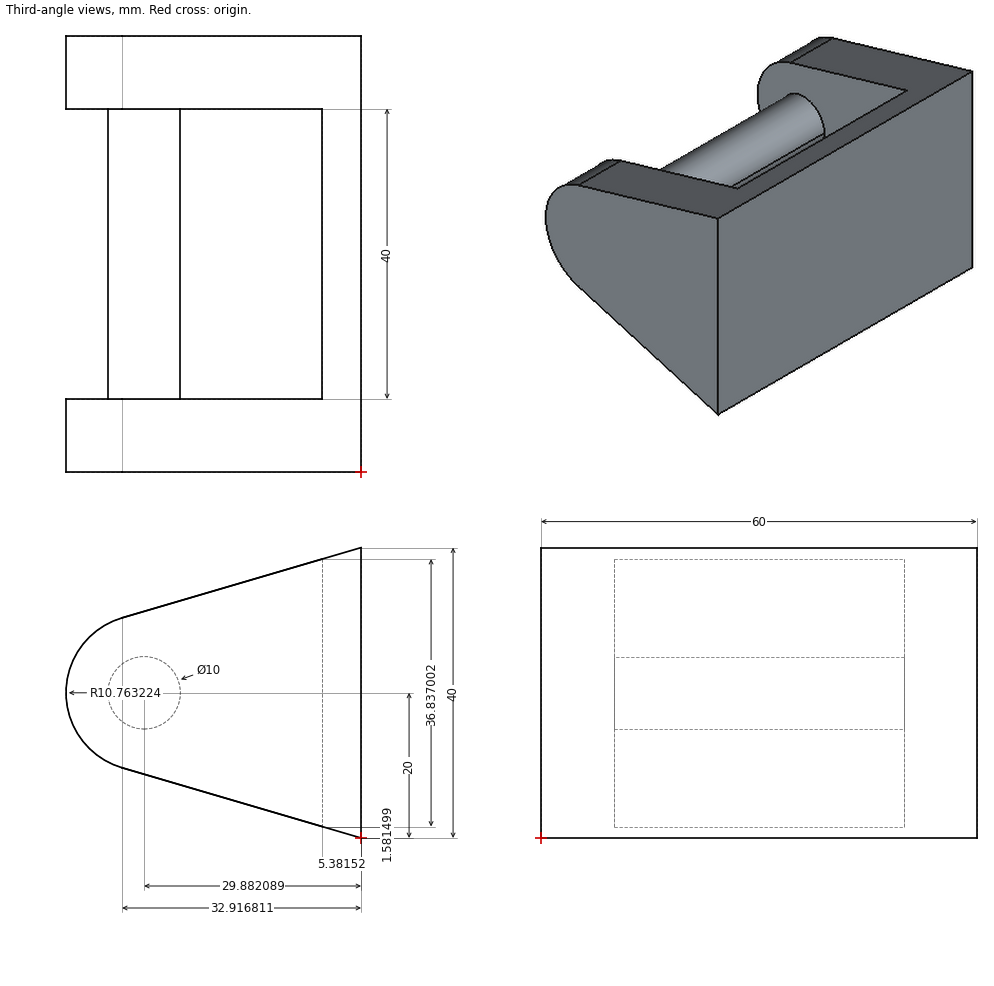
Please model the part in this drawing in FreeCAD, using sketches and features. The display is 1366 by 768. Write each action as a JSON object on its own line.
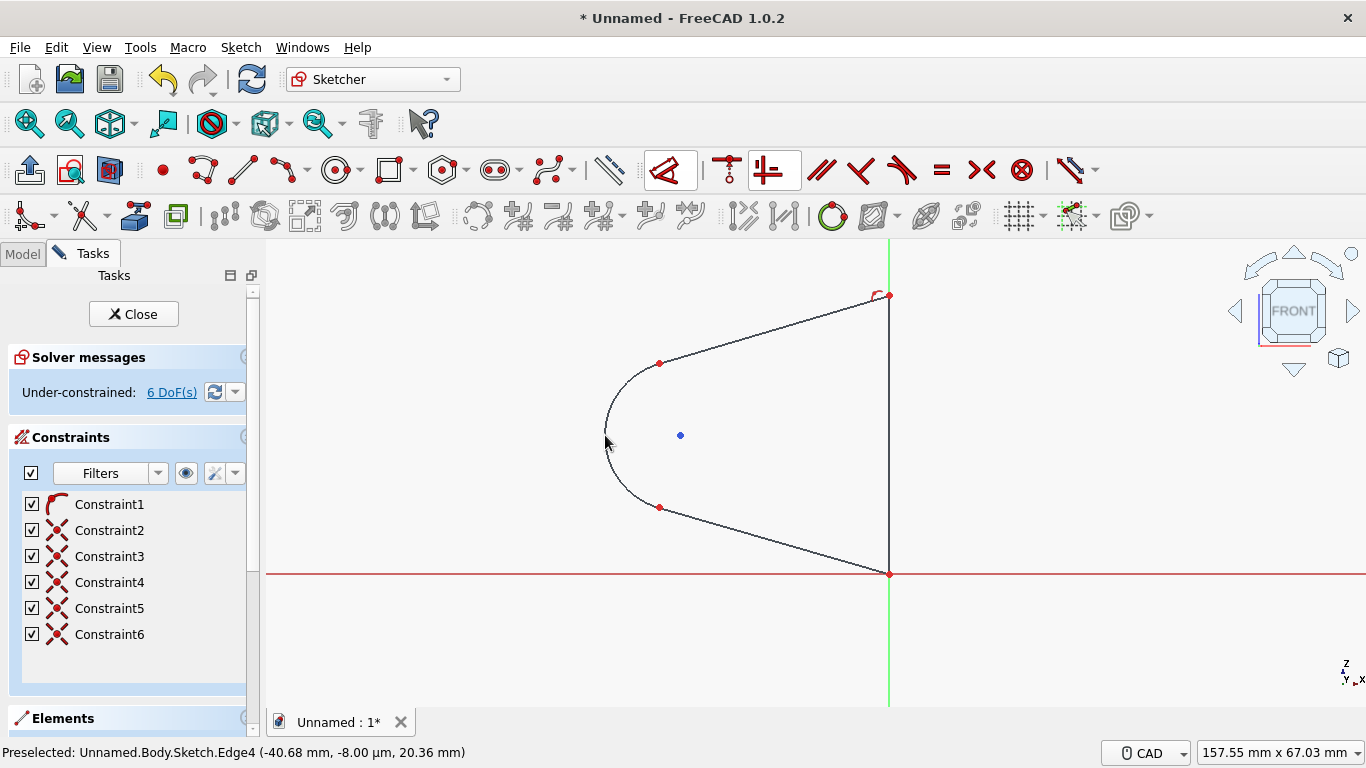
{"action": "left_click", "coordinate": [728, 344]}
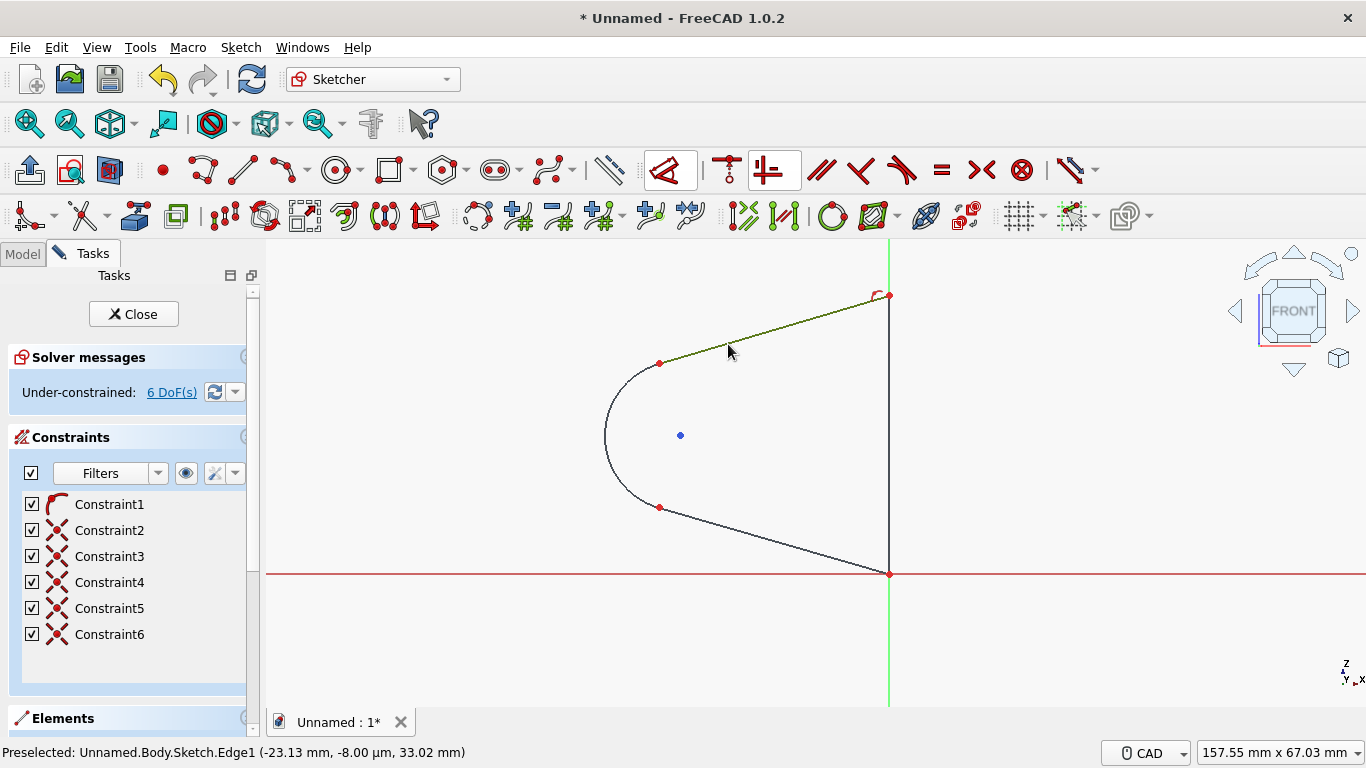
{"action": "left_click", "coordinate": [615, 399]}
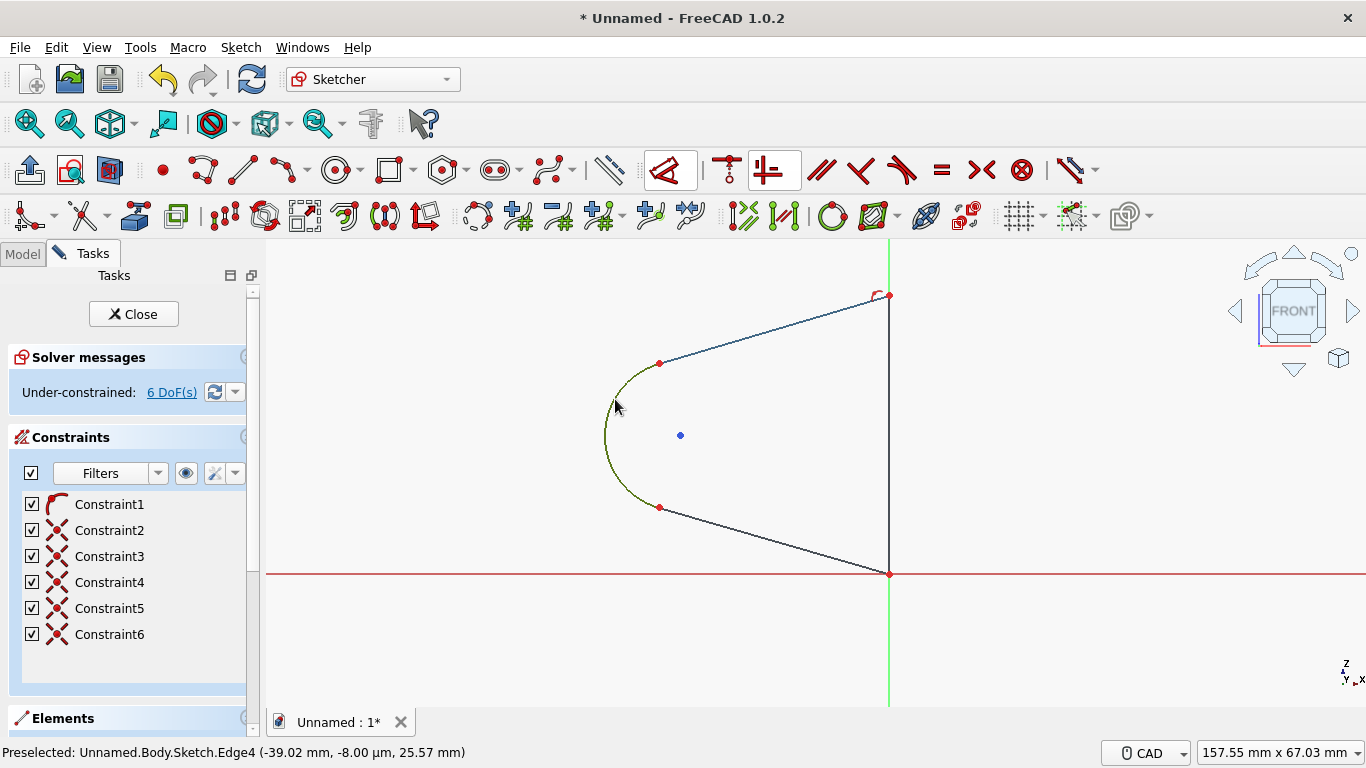
{"action": "left_click", "coordinate": [902, 170]}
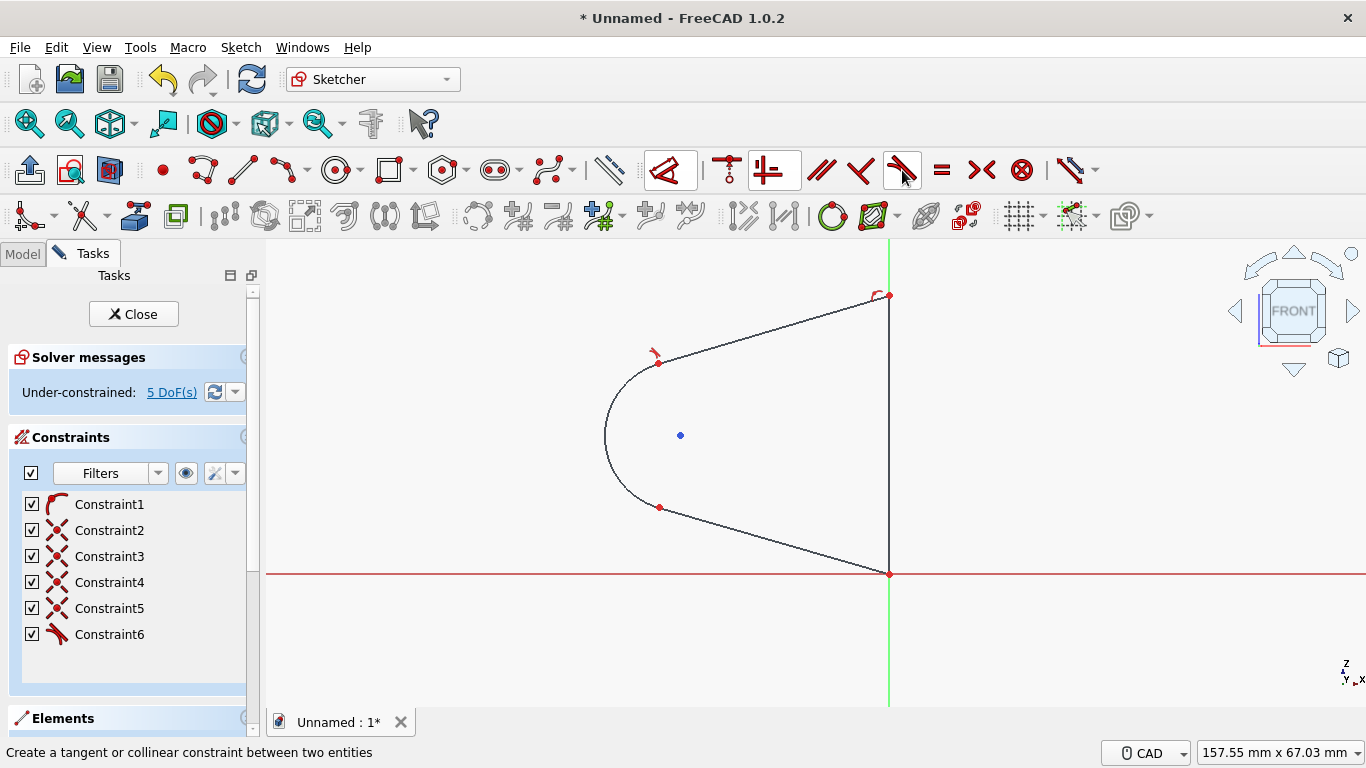
{"action": "left_click", "coordinate": [820, 554]}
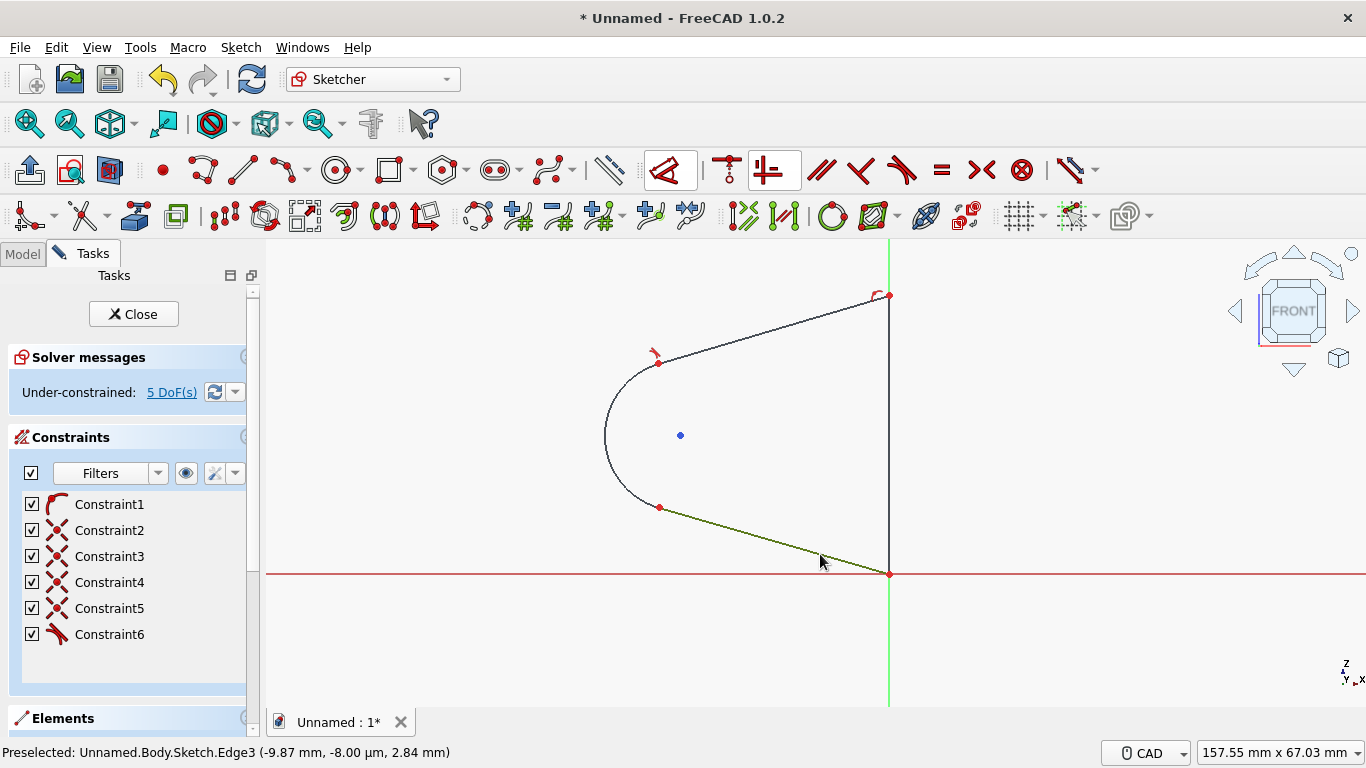
{"action": "left_click", "coordinate": [615, 399]}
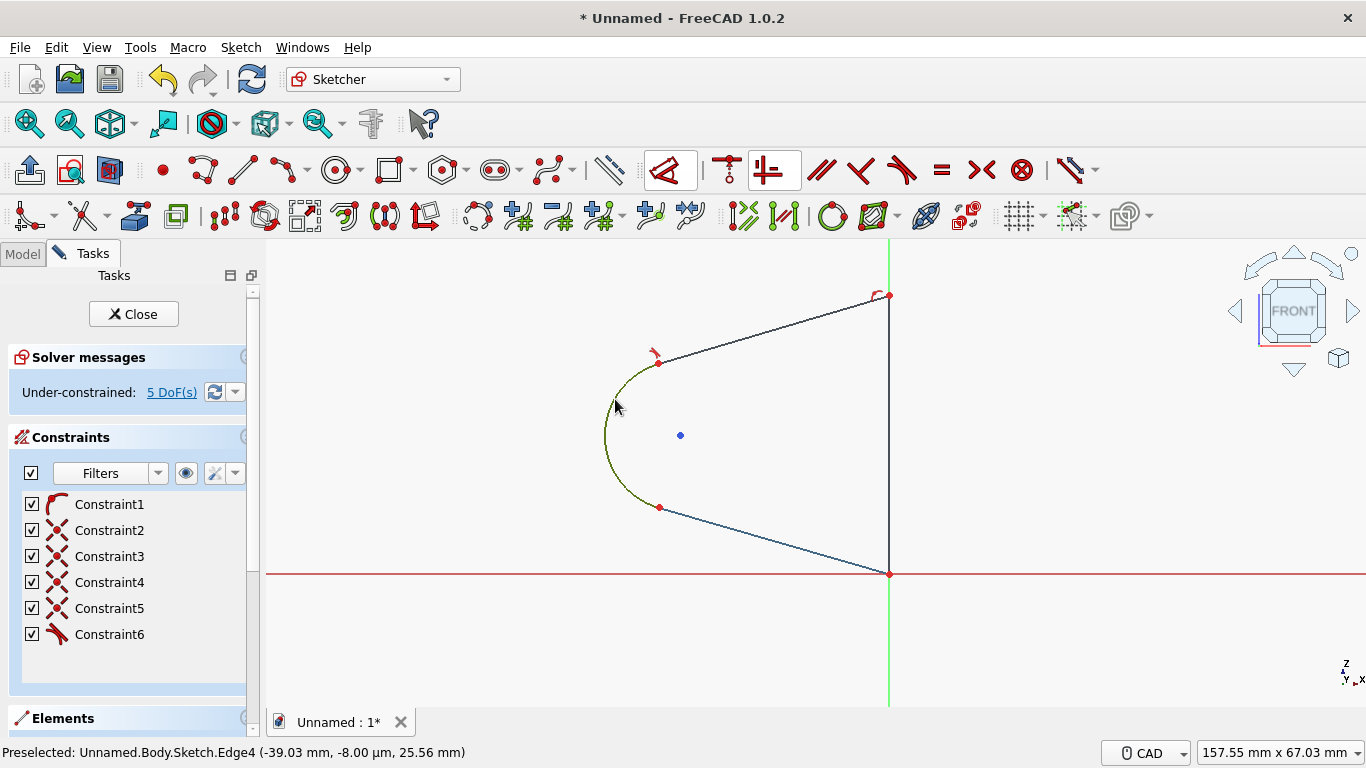
{"action": "left_click", "coordinate": [902, 170]}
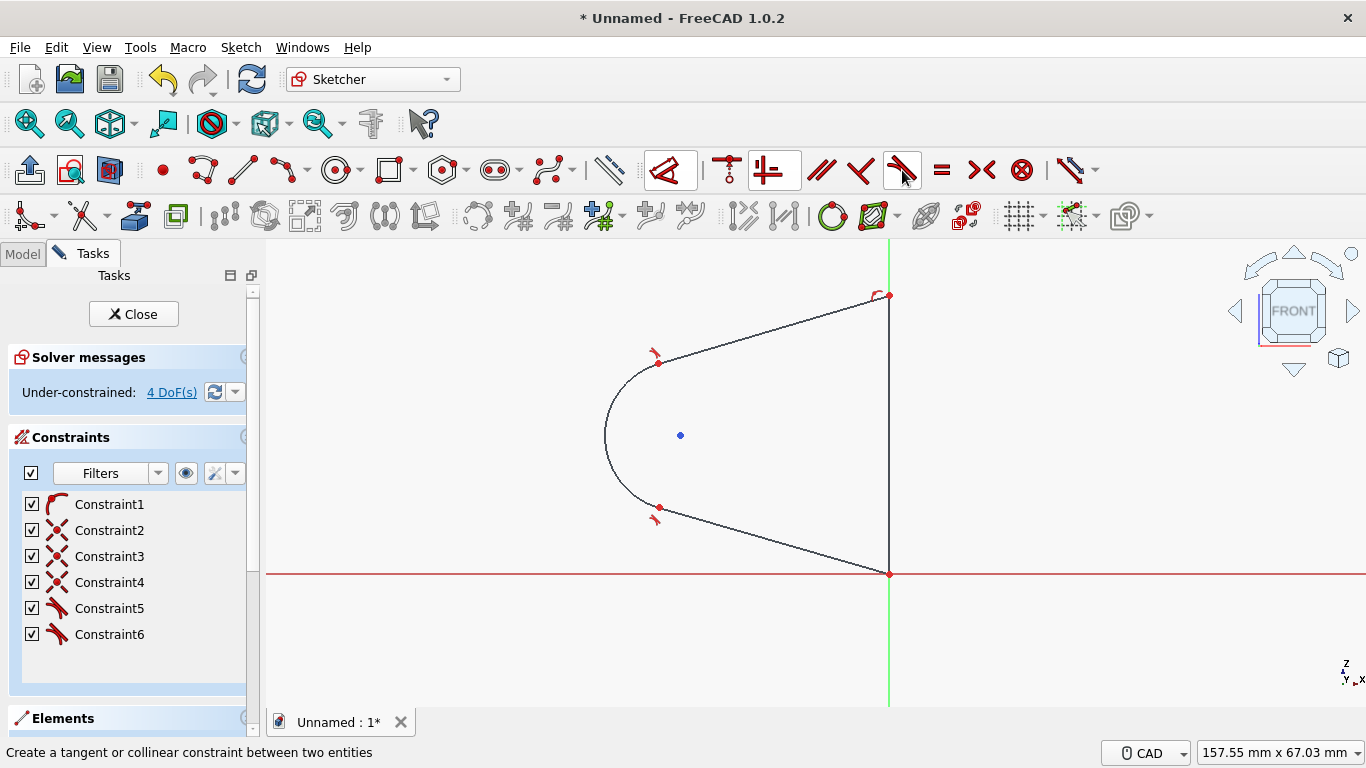
{"action": "left_click", "coordinate": [664, 170]}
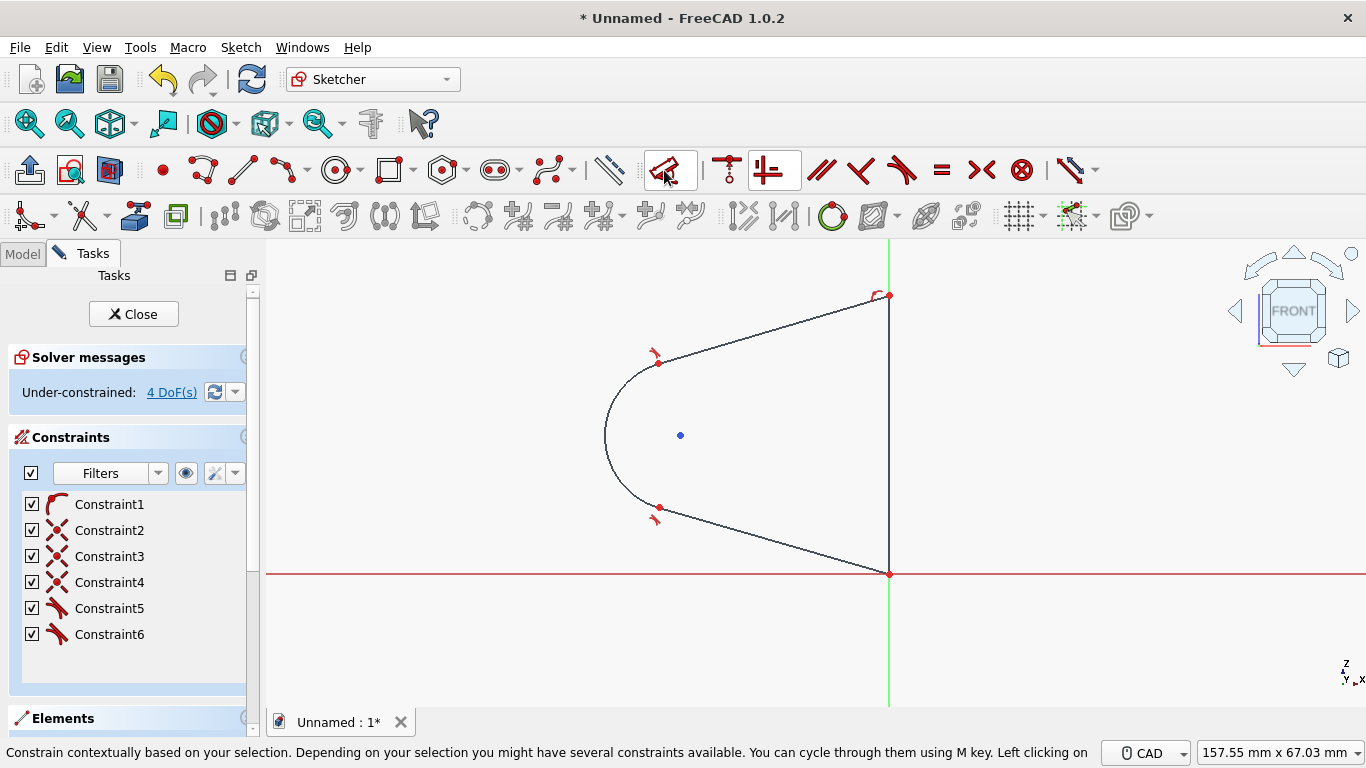
{"action": "left_click", "coordinate": [615, 399]}
{"action": "left_click", "coordinate": [587, 383]}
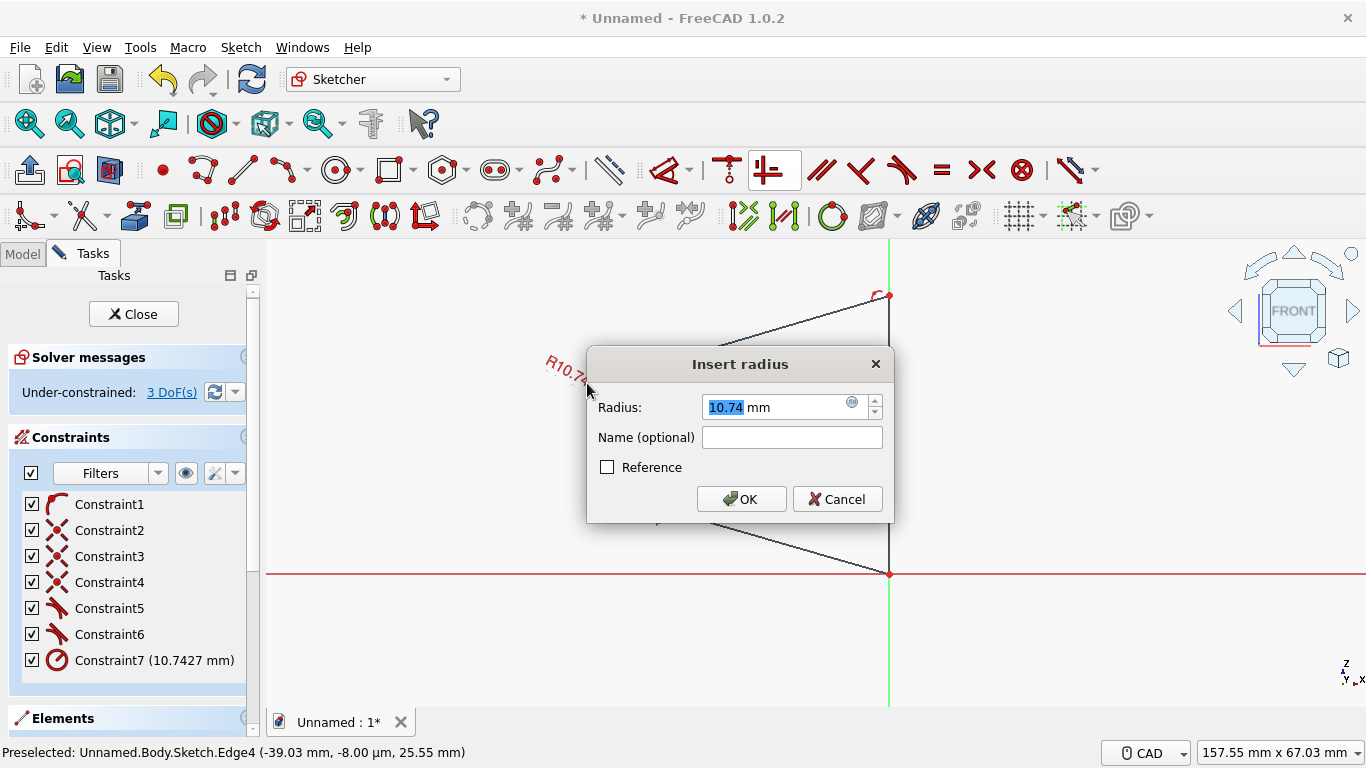
{"action": "type", "text": "10.763224"}
{"action": "key", "text": "Return"}